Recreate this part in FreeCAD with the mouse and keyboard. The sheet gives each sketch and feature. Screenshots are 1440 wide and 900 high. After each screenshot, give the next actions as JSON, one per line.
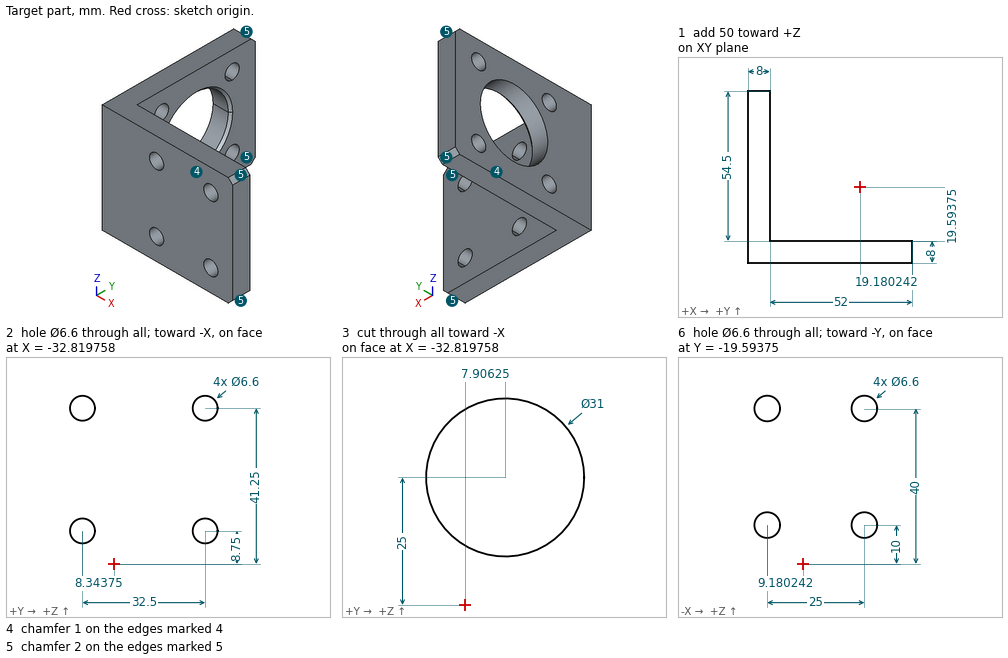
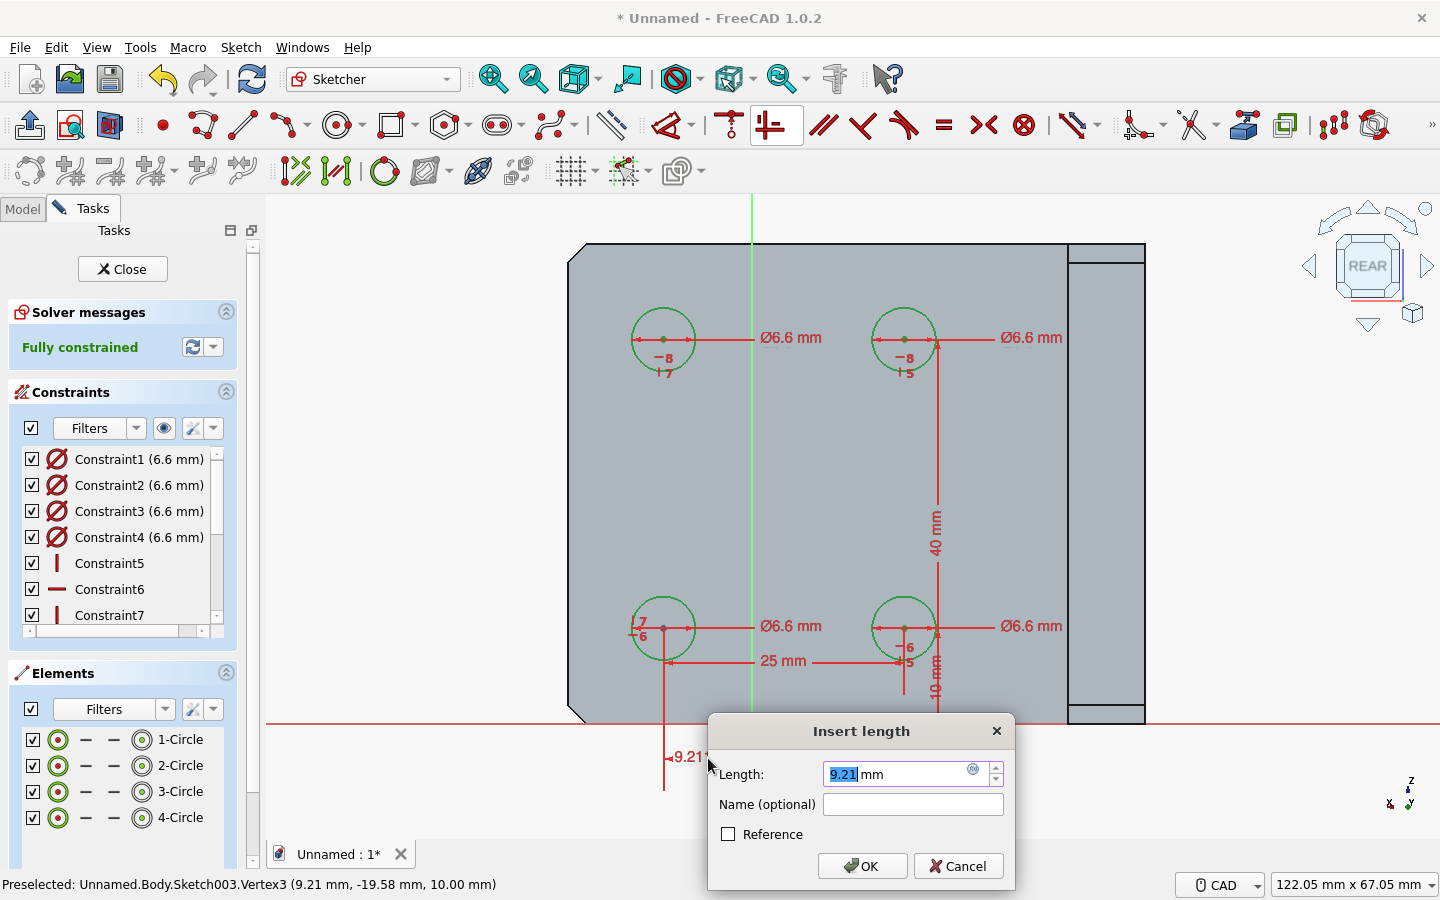
{"action": "type", "text": "9.180242"}
{"action": "key", "text": "Return"}
{"action": "key", "text": "Escape"}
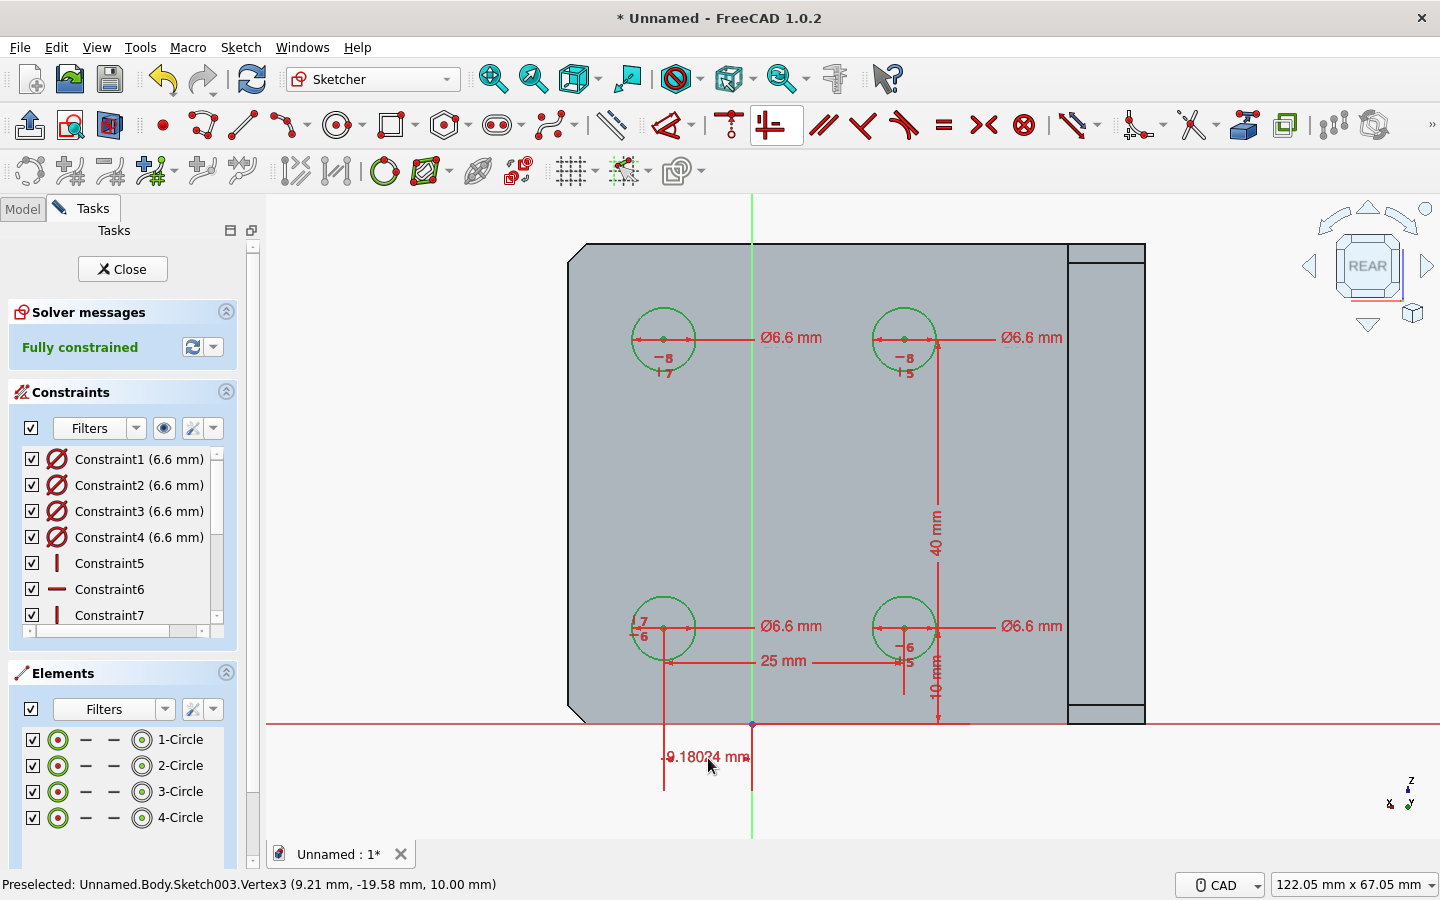
{"action": "left_click", "coordinate": [123, 269]}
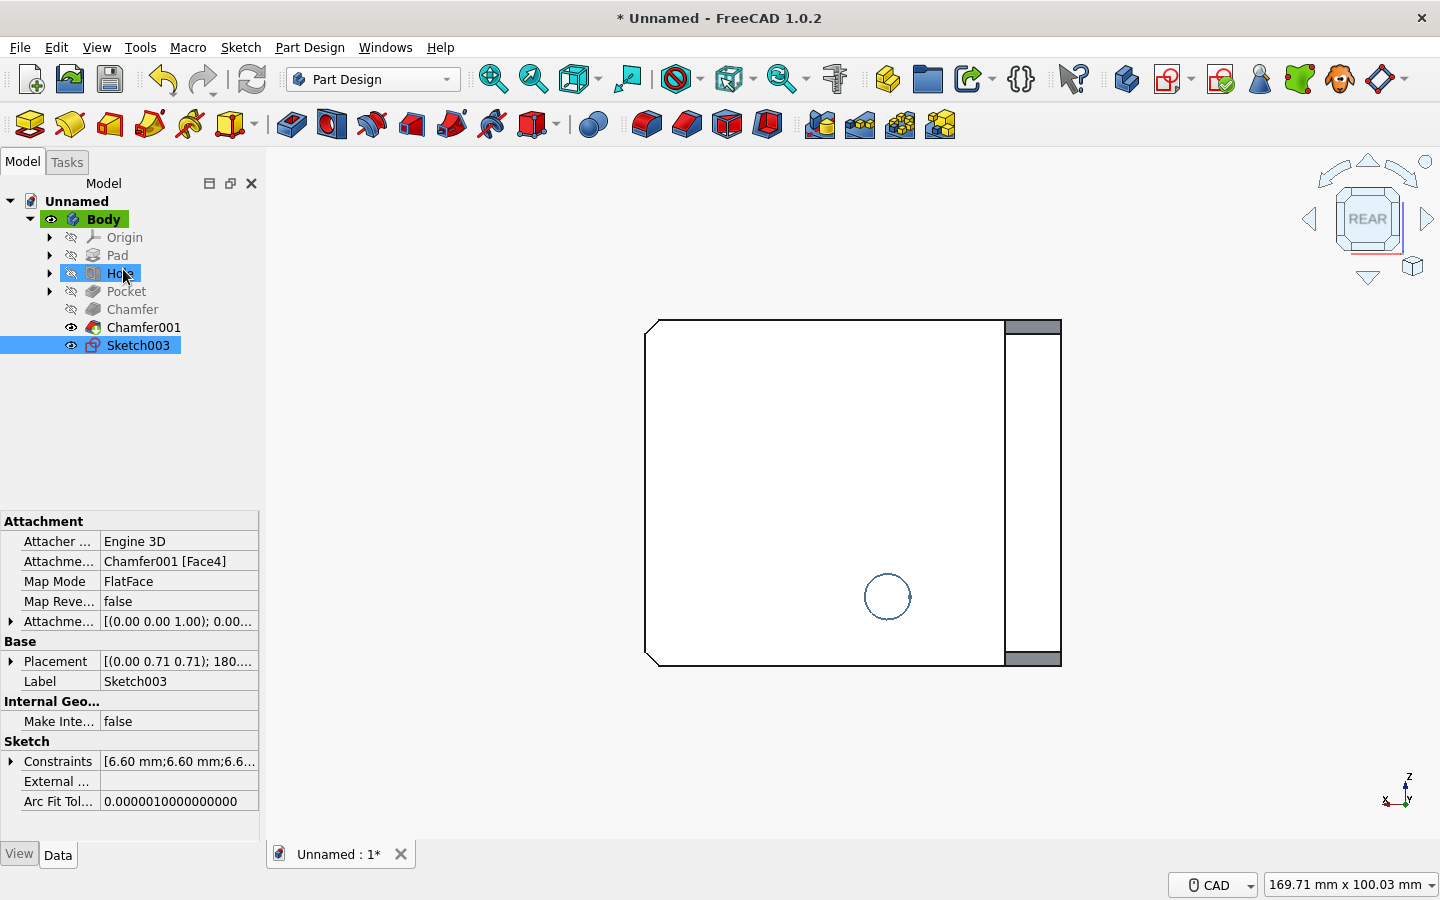
{"action": "left_click", "coordinate": [332, 124]}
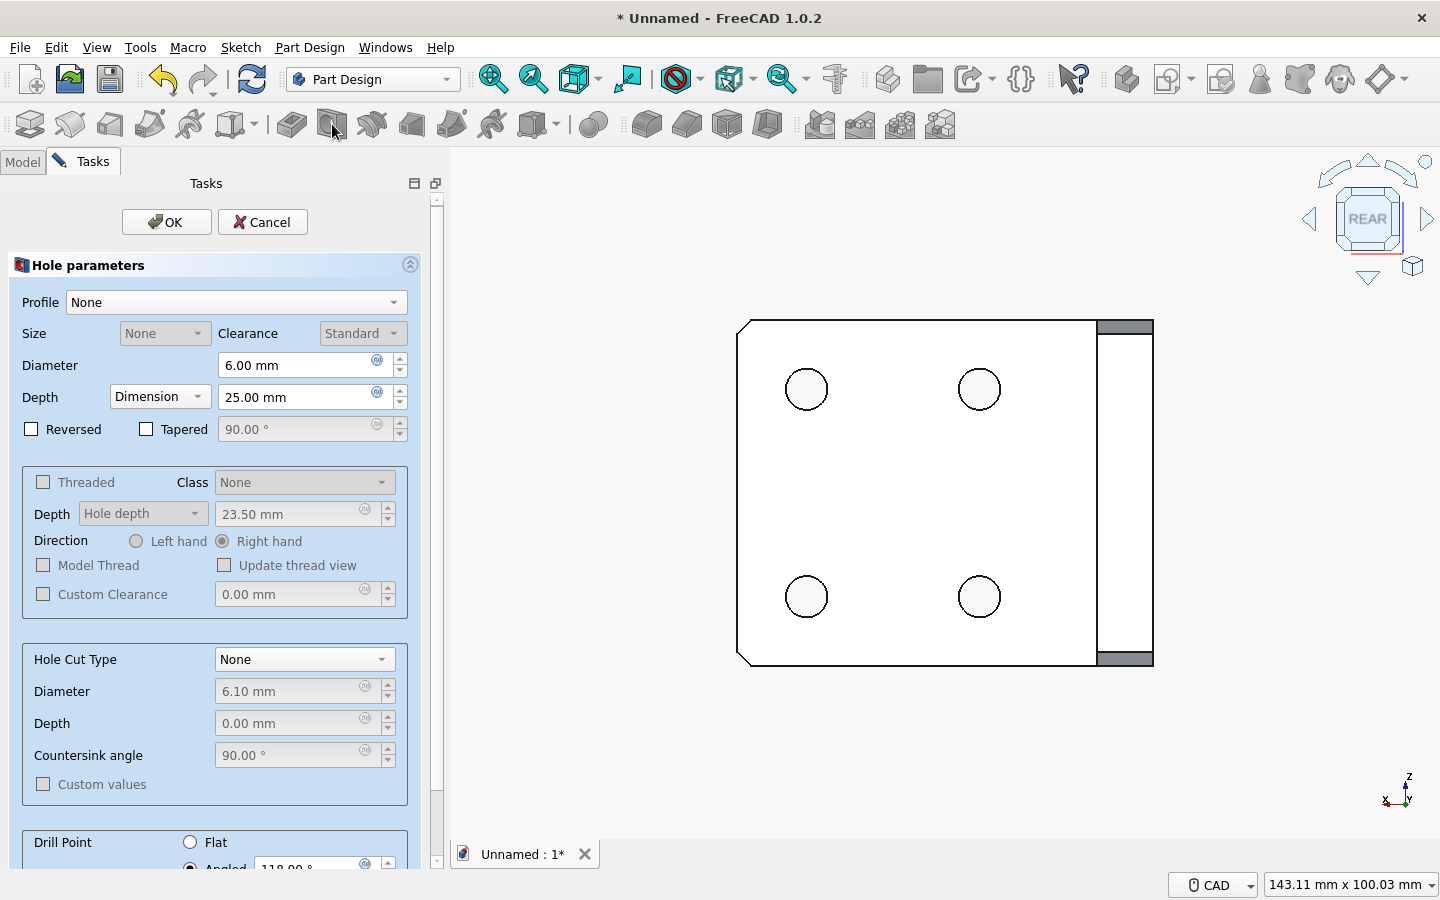
{"action": "triple_click", "coordinate": [305, 365]}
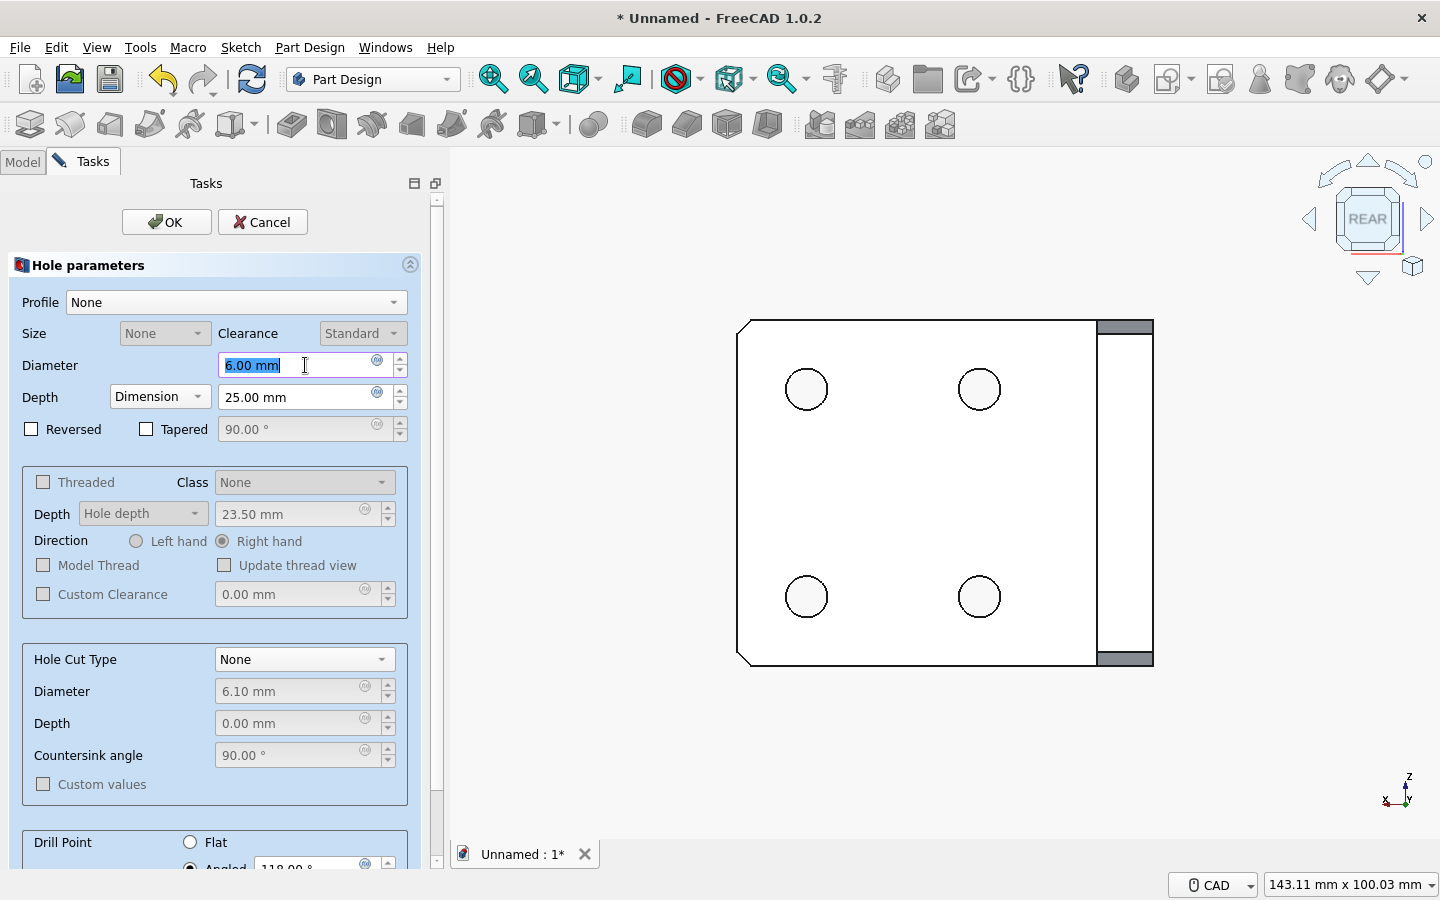
{"action": "type", "text": "6.6"}
{"action": "key", "text": "Tab"}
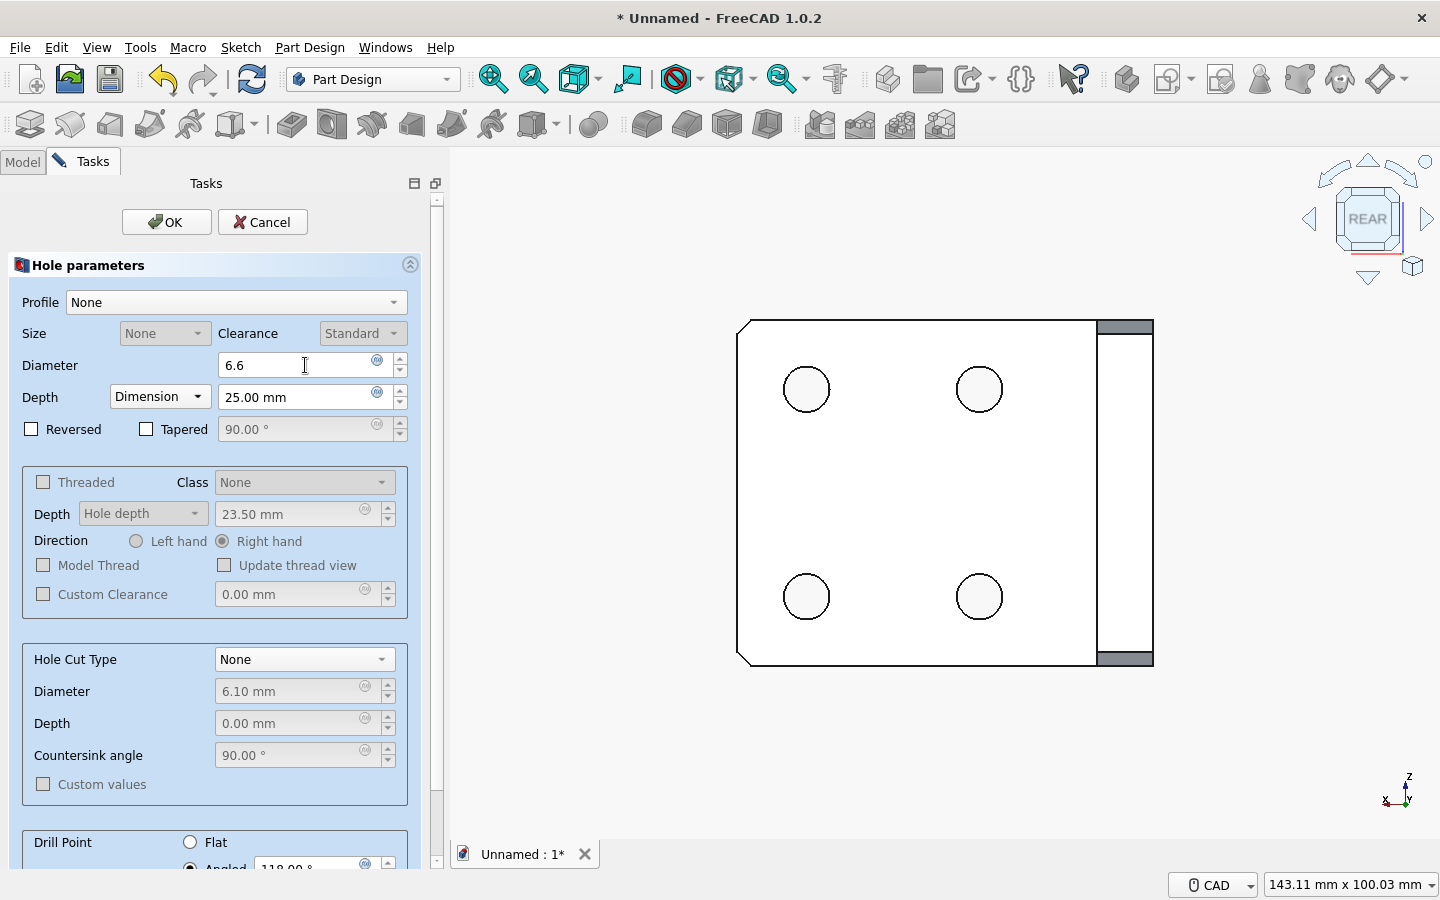
{"action": "left_click", "coordinate": [161, 396]}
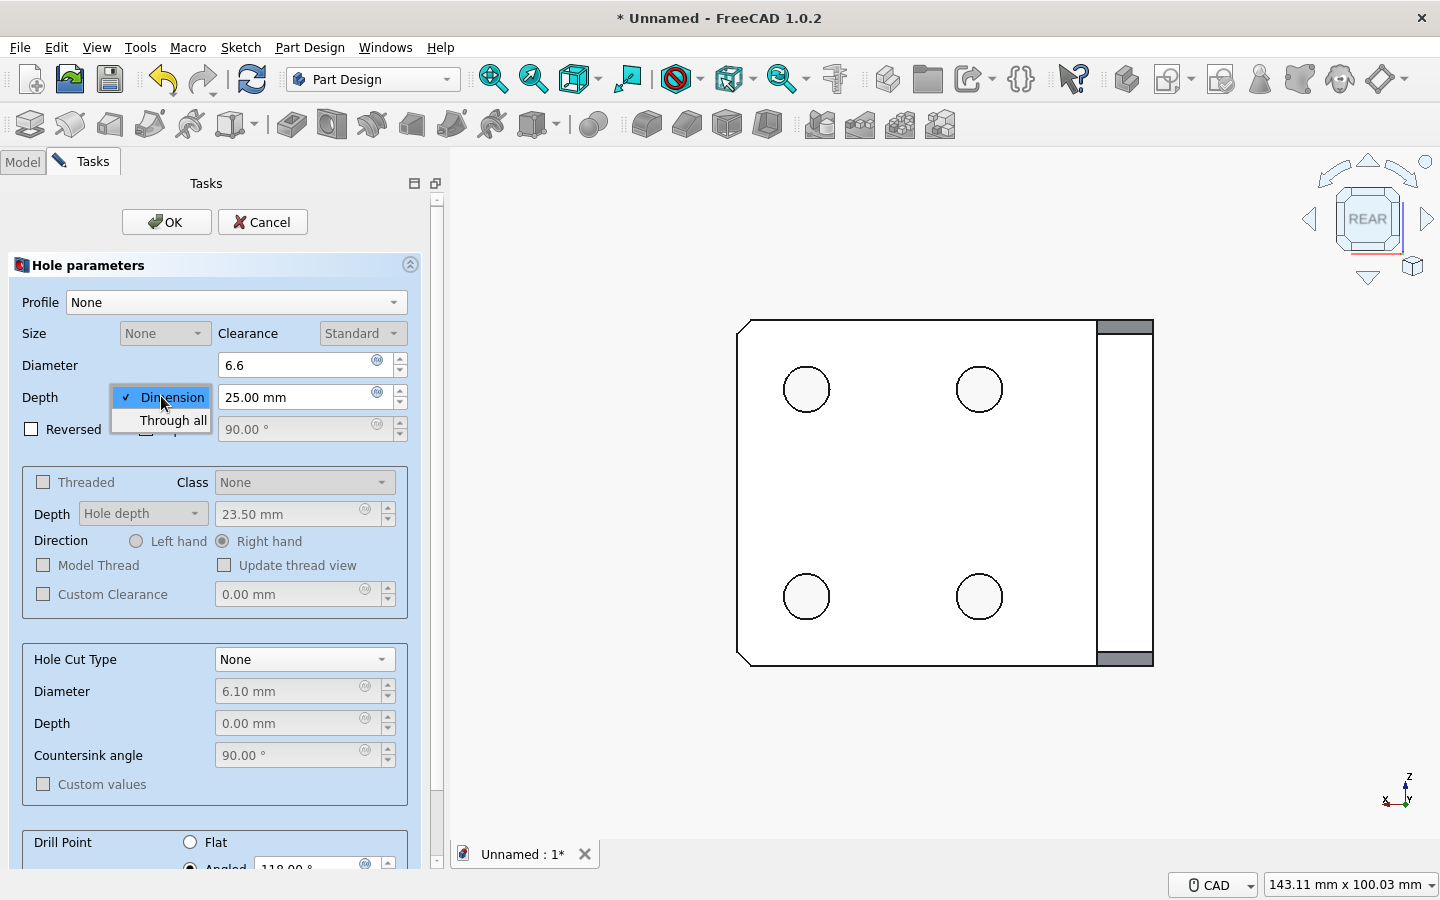
{"action": "left_click", "coordinate": [160, 420]}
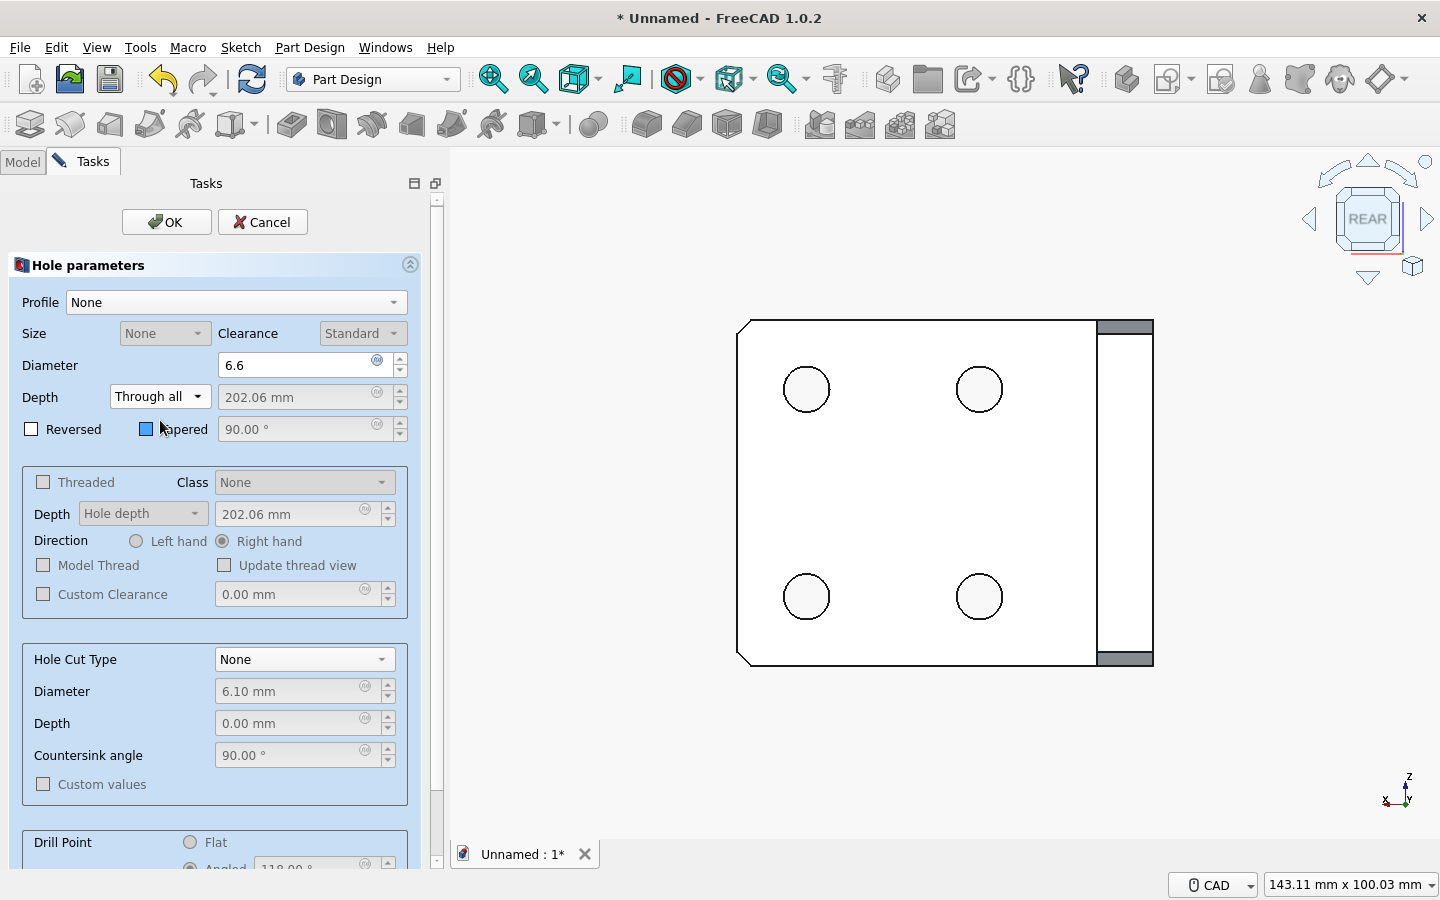
{"action": "left_click", "coordinate": [167, 222]}